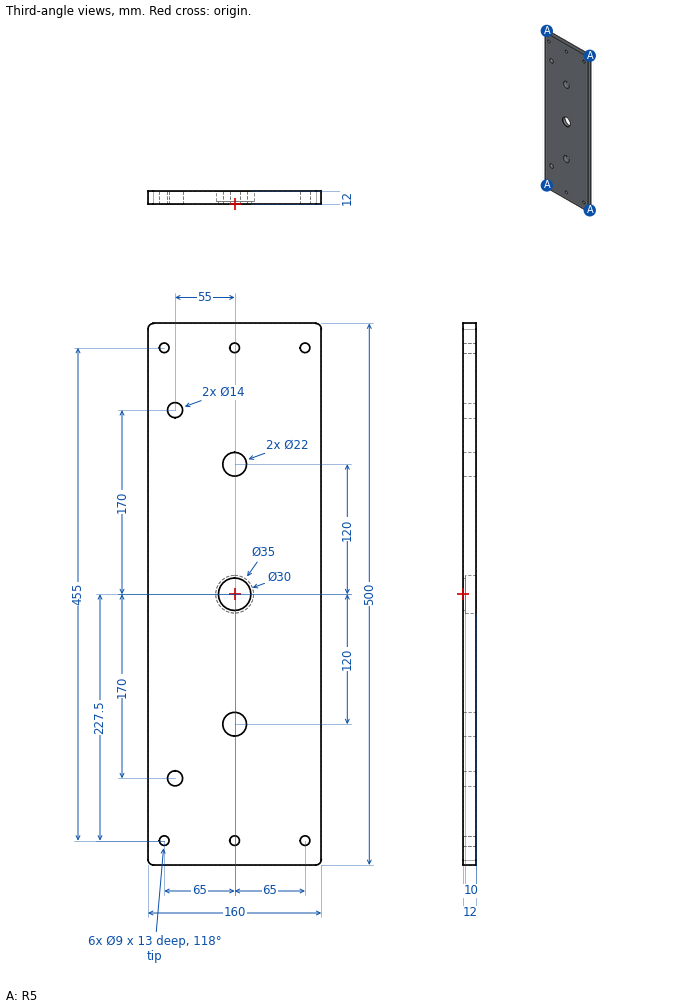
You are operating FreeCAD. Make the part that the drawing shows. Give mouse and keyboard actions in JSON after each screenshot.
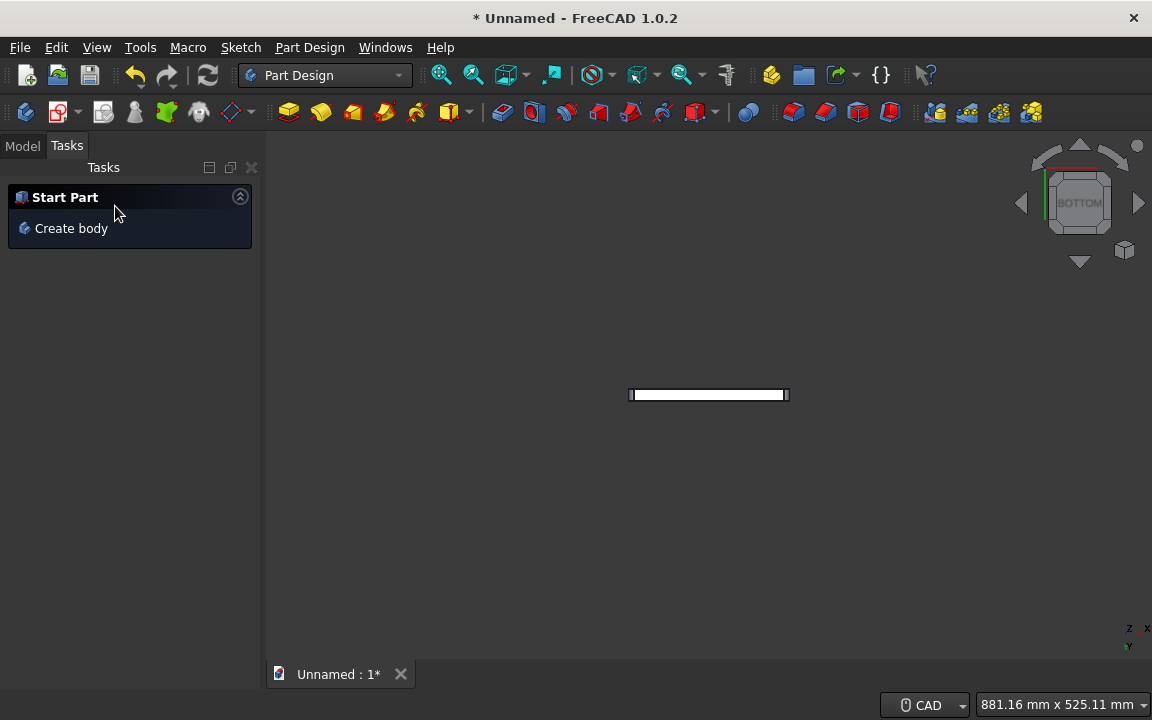
{"action": "key", "text": "0"}